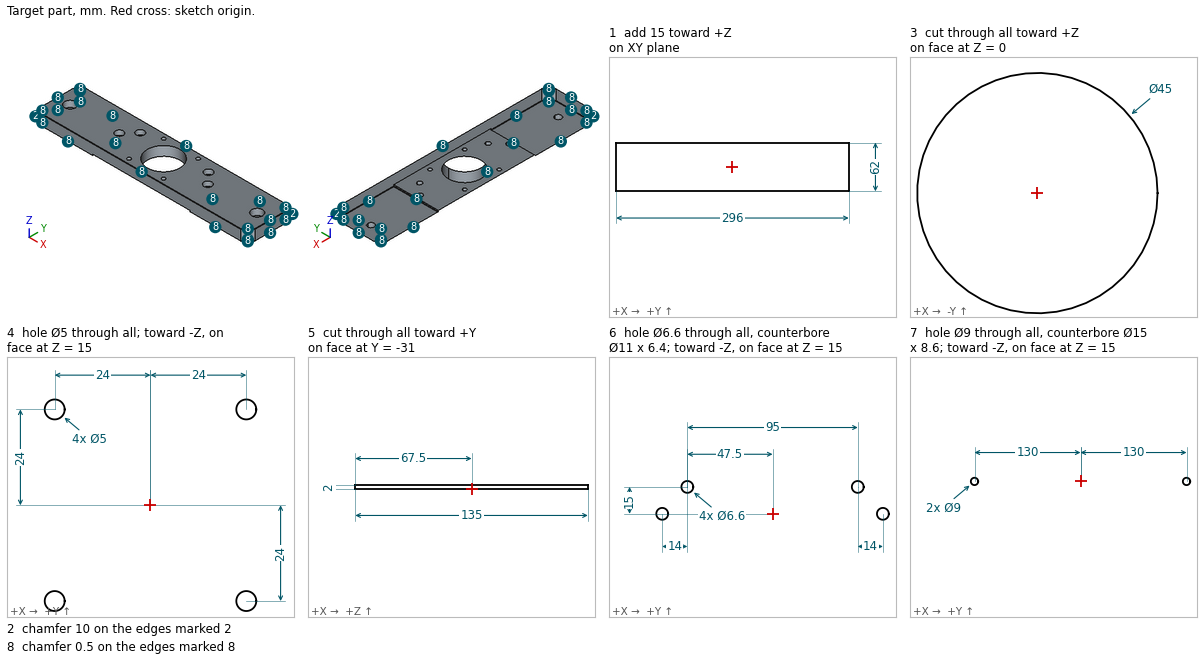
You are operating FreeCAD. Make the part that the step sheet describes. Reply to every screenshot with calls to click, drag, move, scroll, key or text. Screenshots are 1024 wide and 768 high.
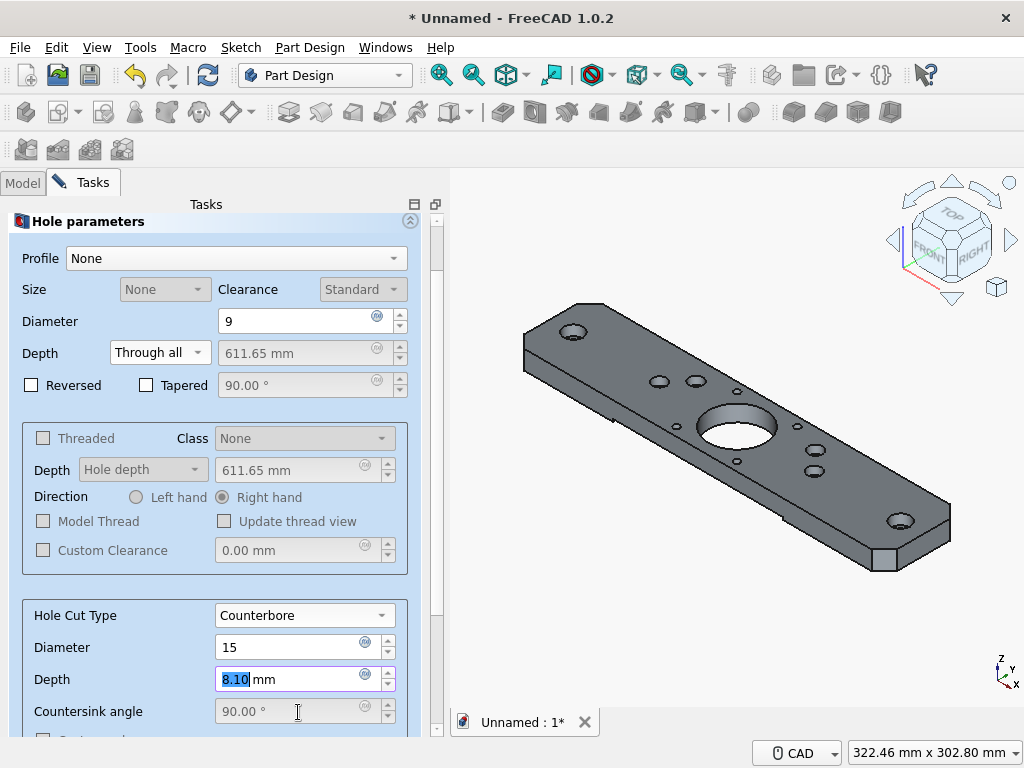
text(8.6)
key(Tab)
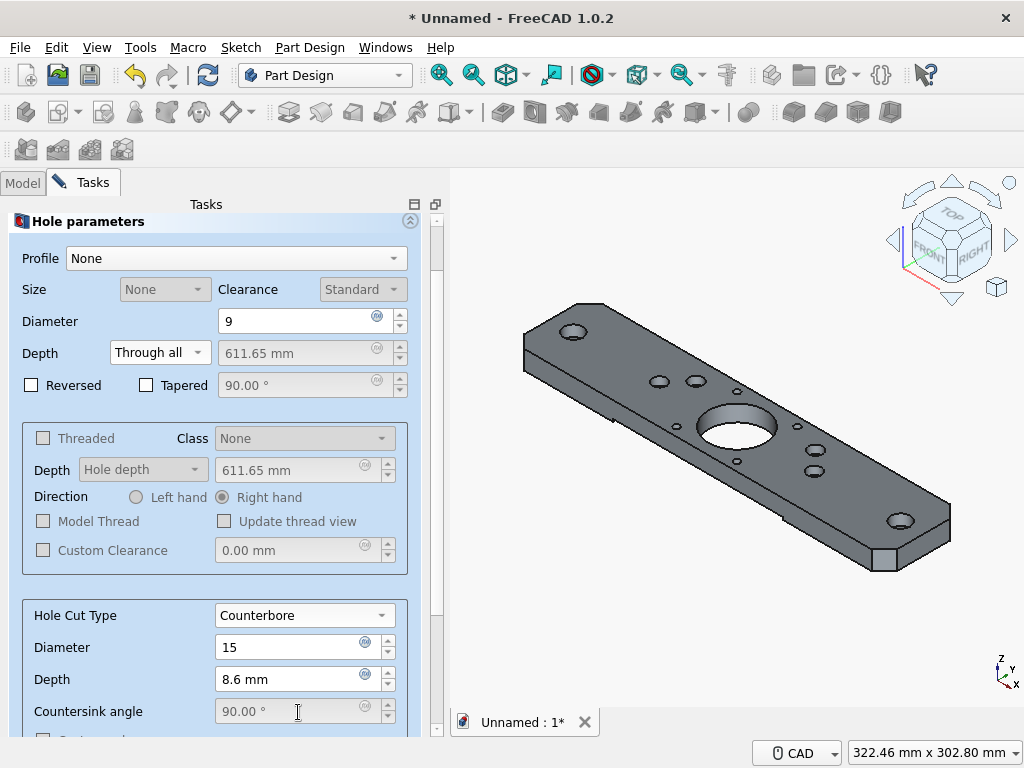
scroll(437, 475, up, 2)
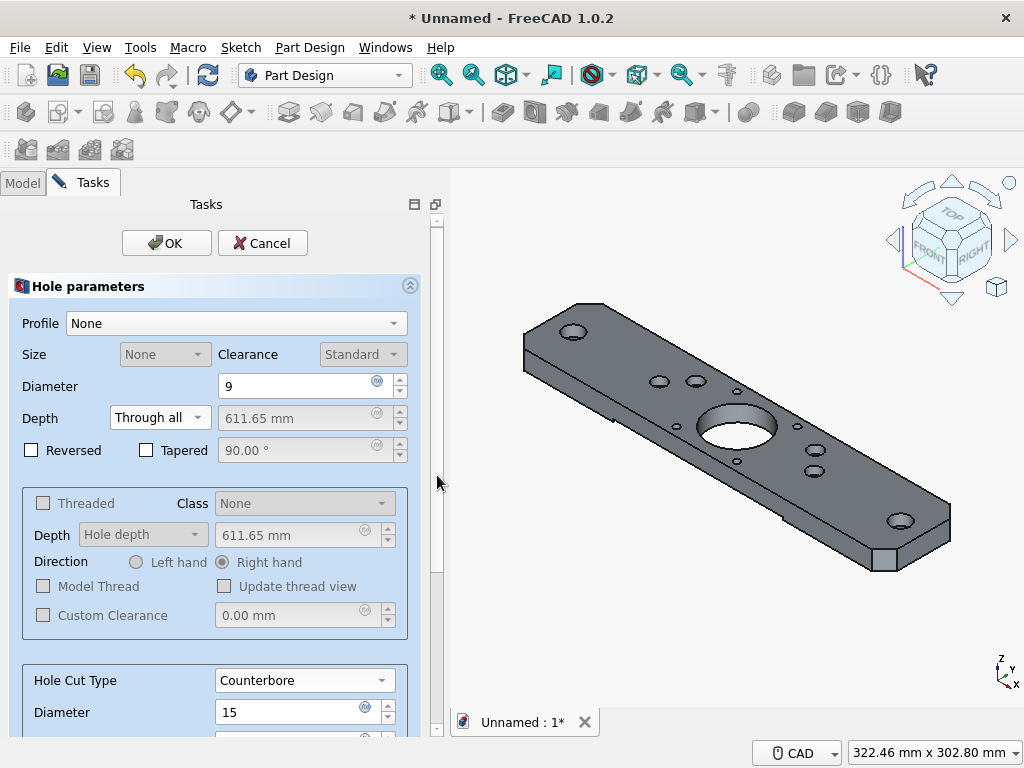
click(167, 243)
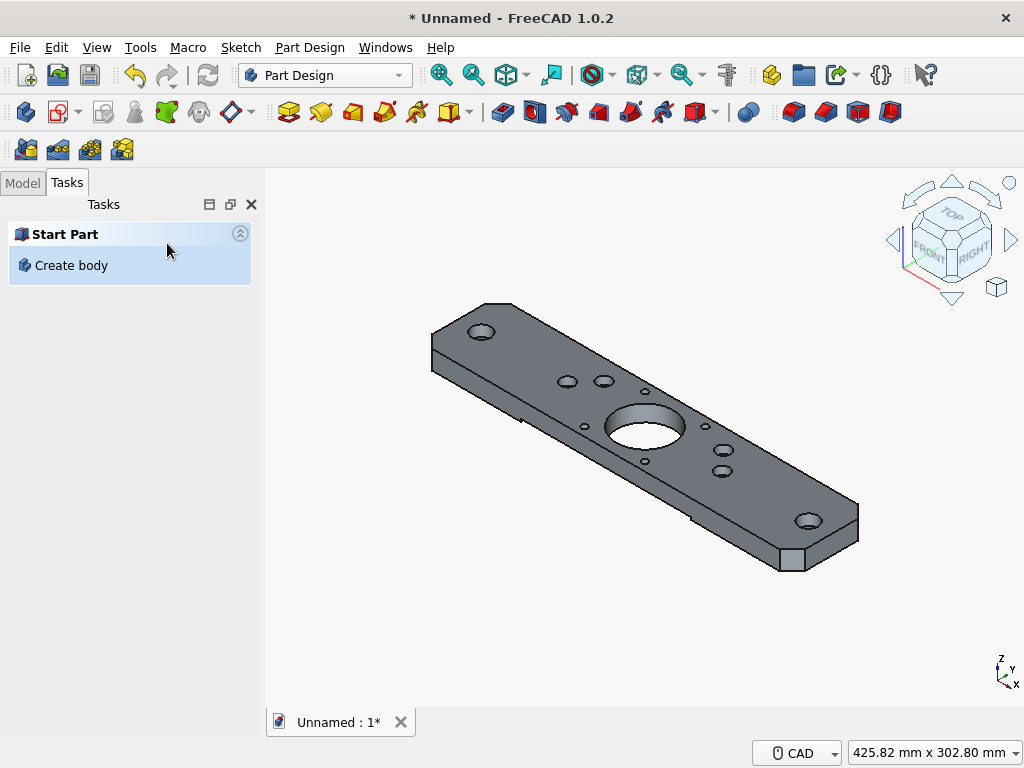
click(831, 533)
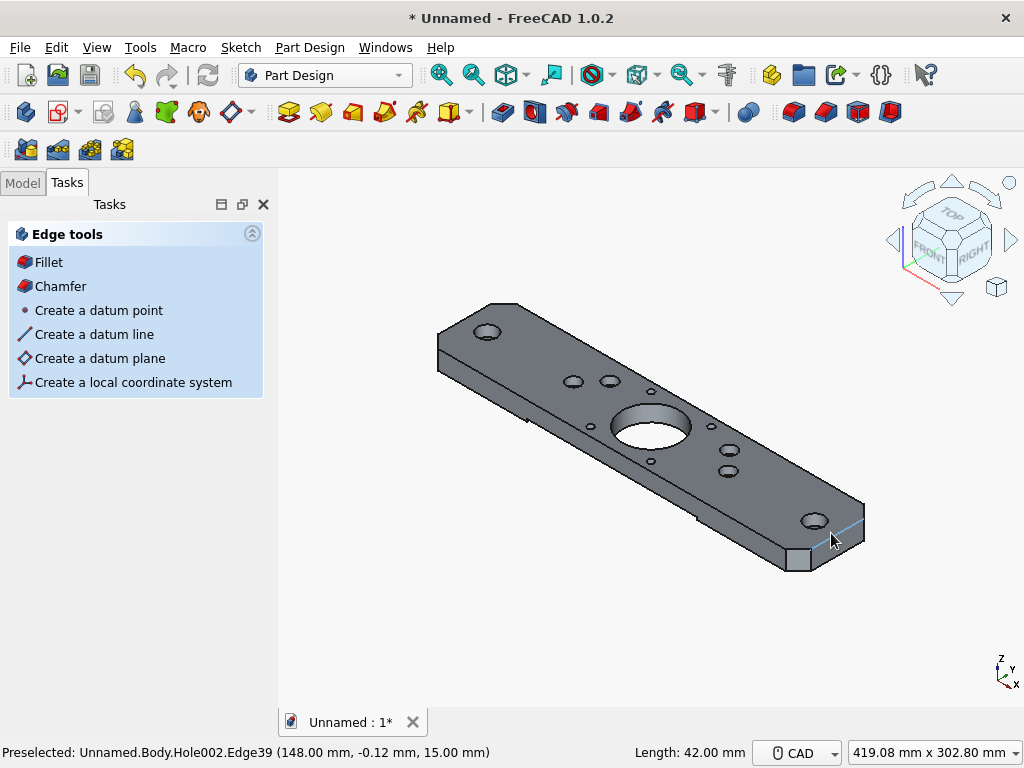
click(612, 448, ctrl)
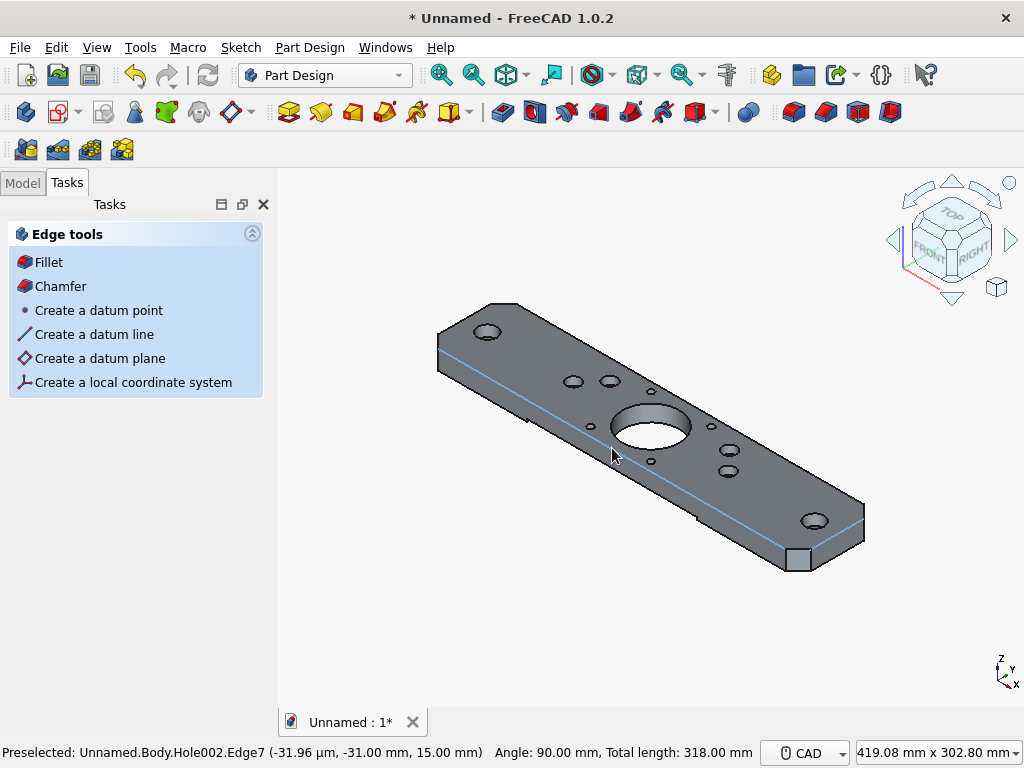
click(438, 339, ctrl)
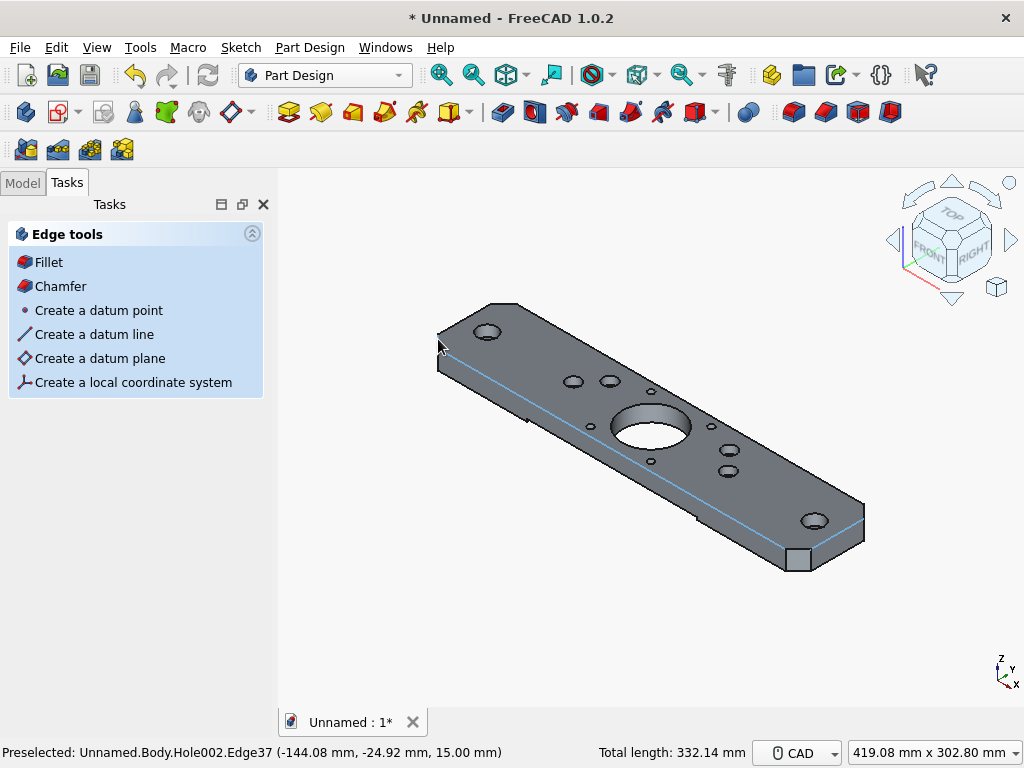
click(798, 548, ctrl)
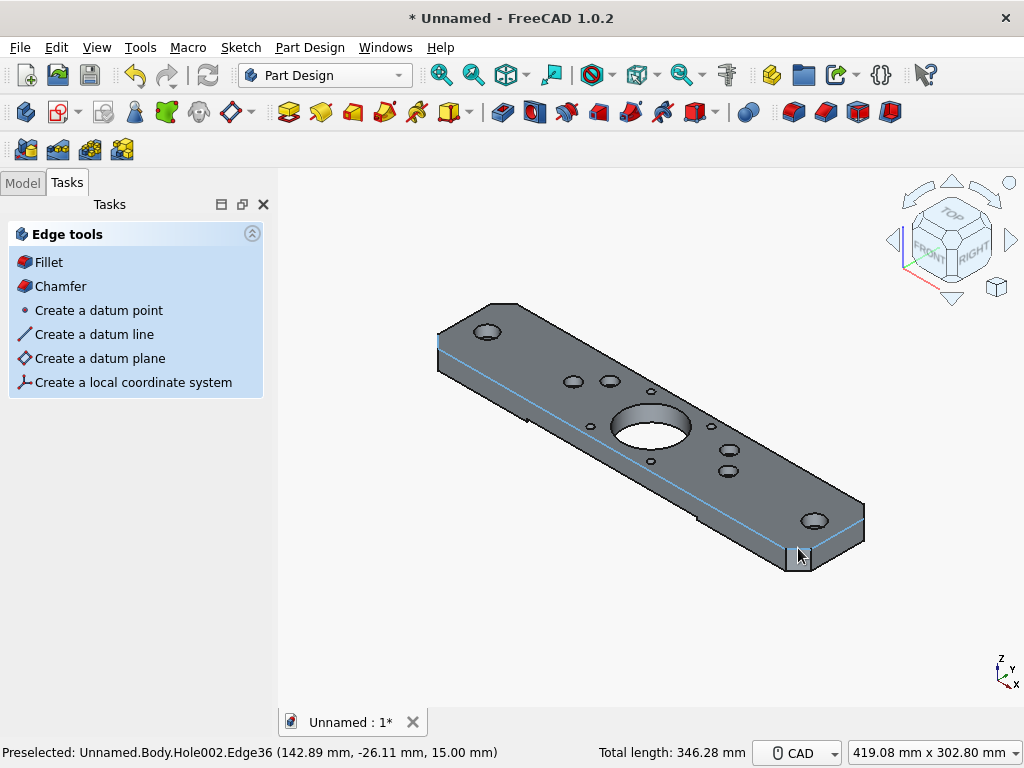
click(864, 508, ctrl)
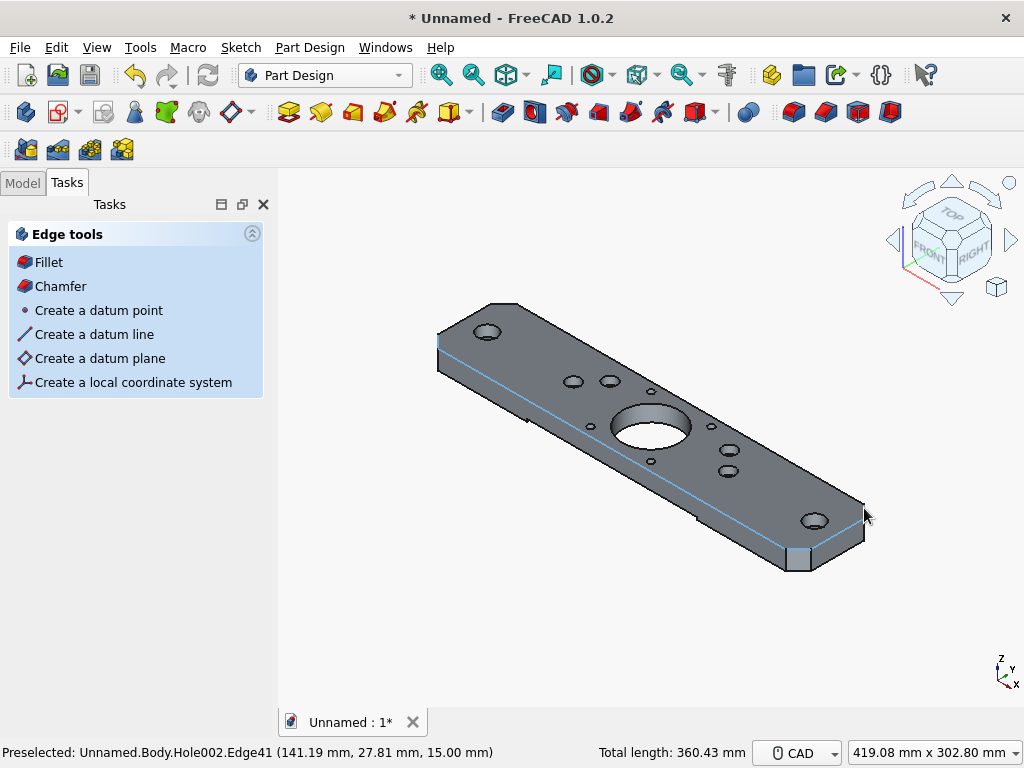
key(2)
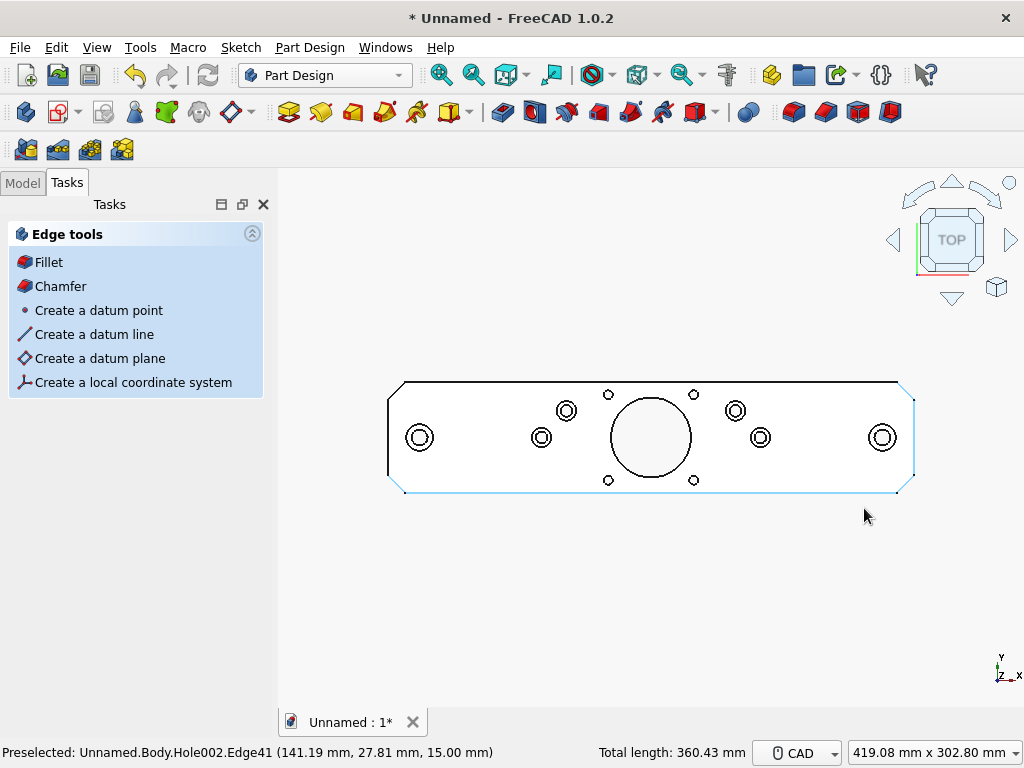
click(651, 381, ctrl)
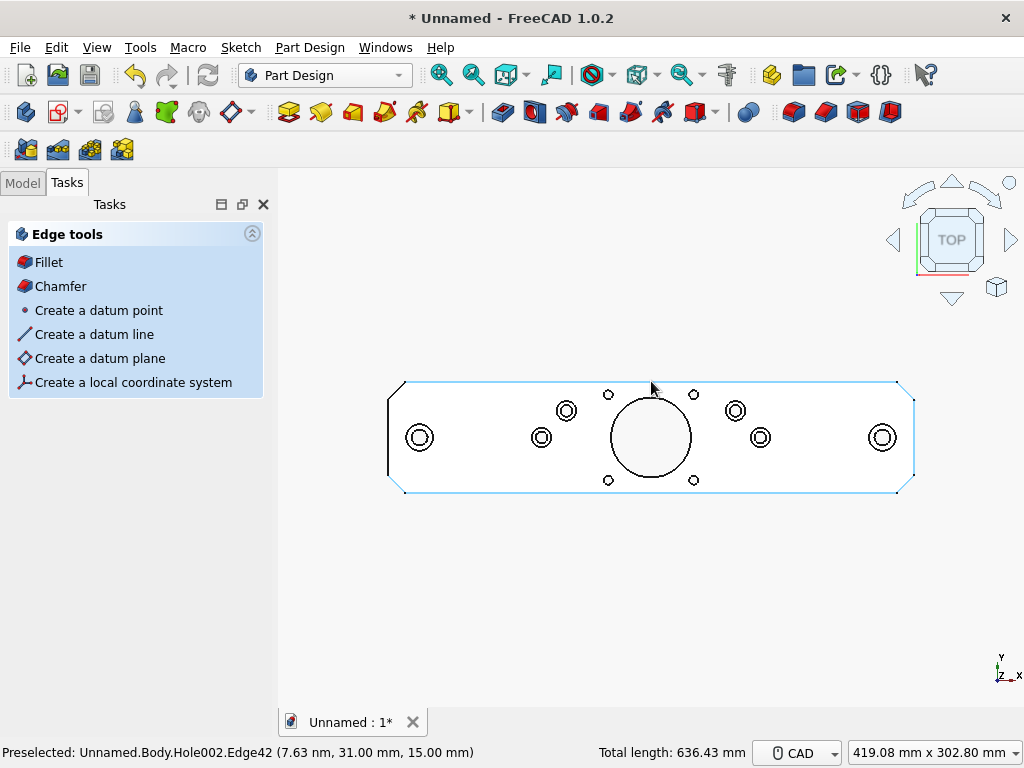
click(388, 436, ctrl)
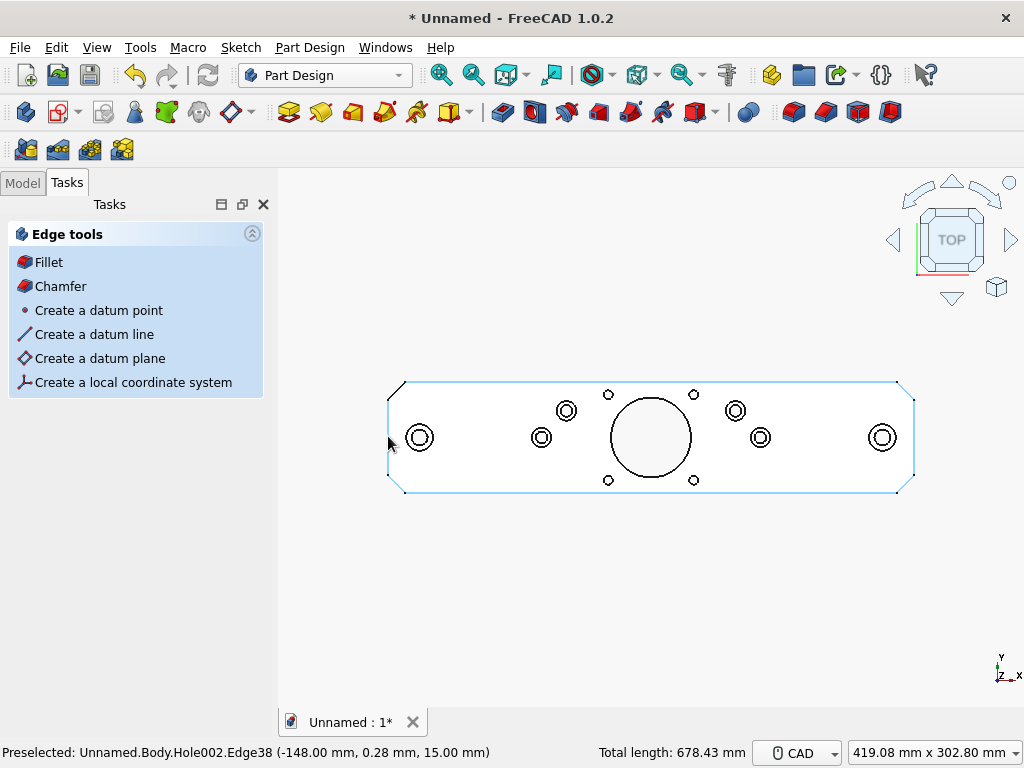
click(396, 390, ctrl)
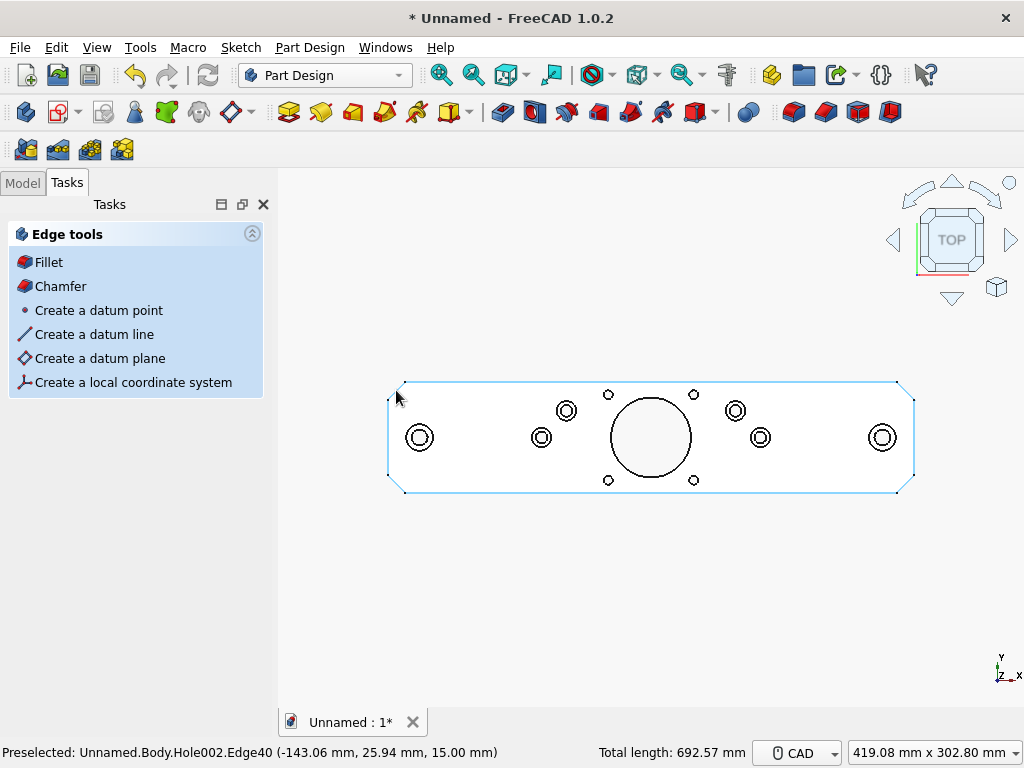
key(0)